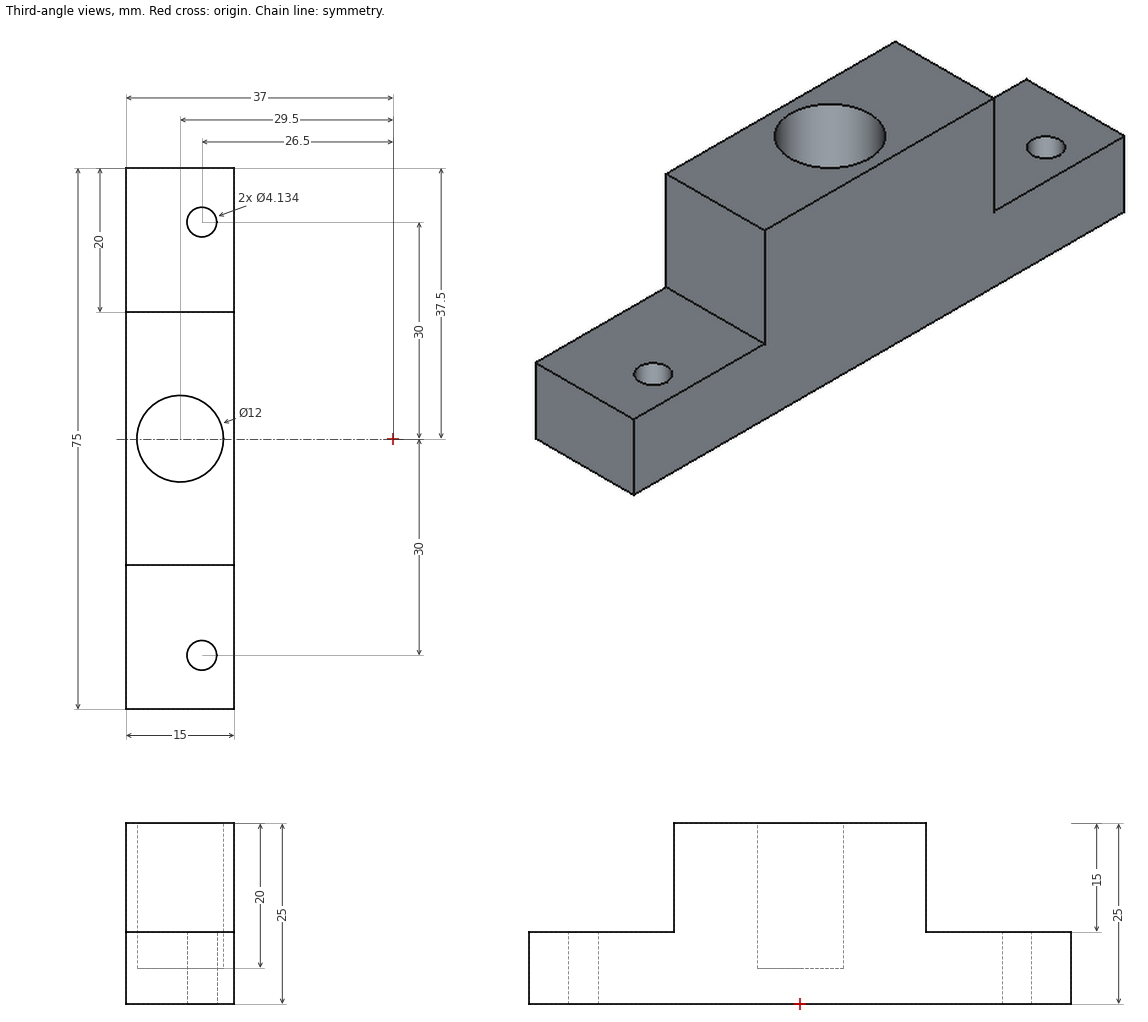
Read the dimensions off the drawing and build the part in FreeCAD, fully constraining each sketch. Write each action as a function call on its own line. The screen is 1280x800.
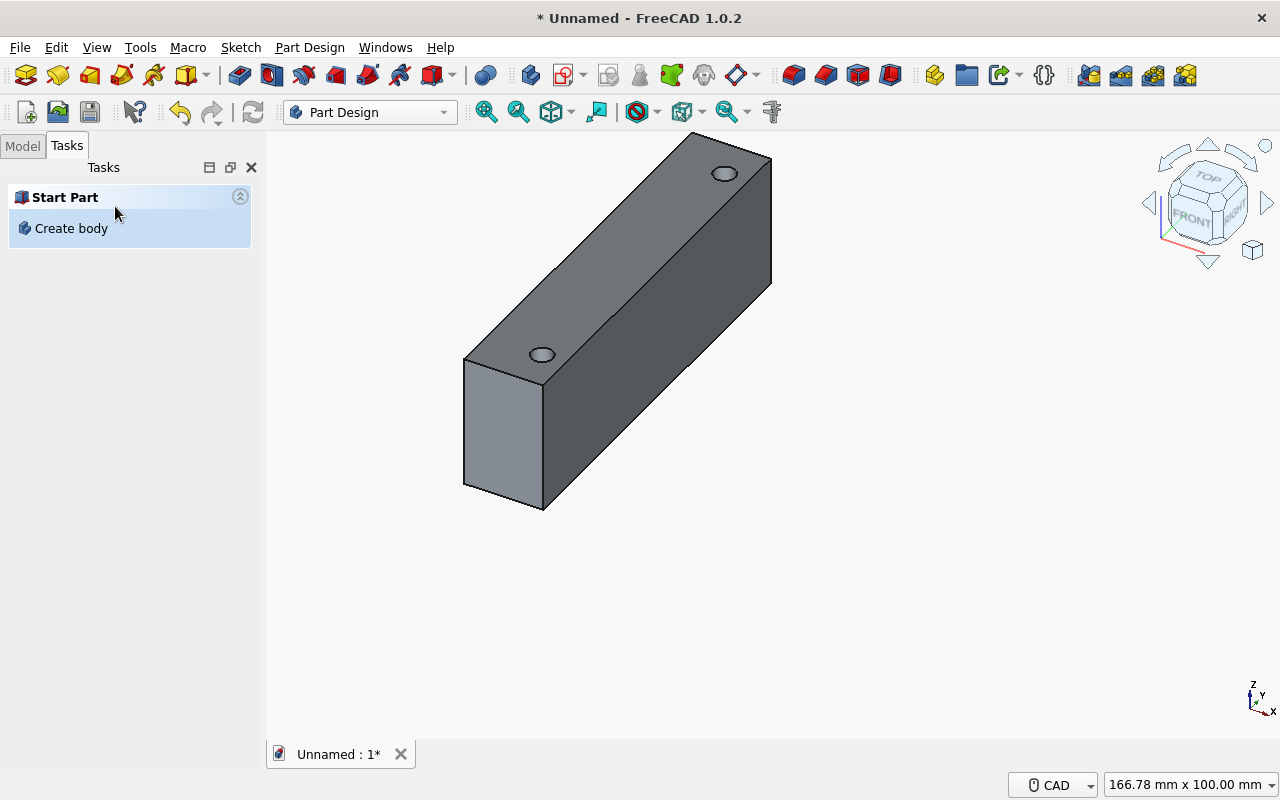
click(650, 226)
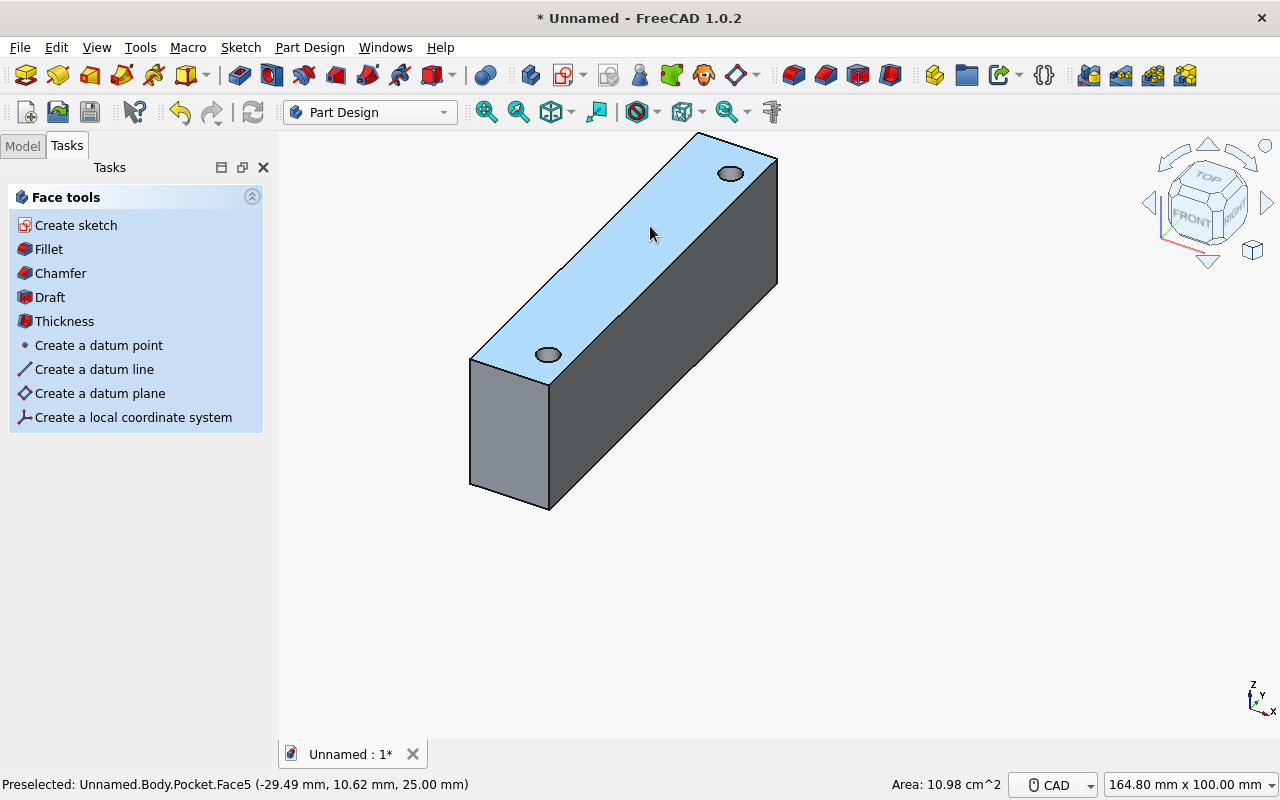
click(564, 76)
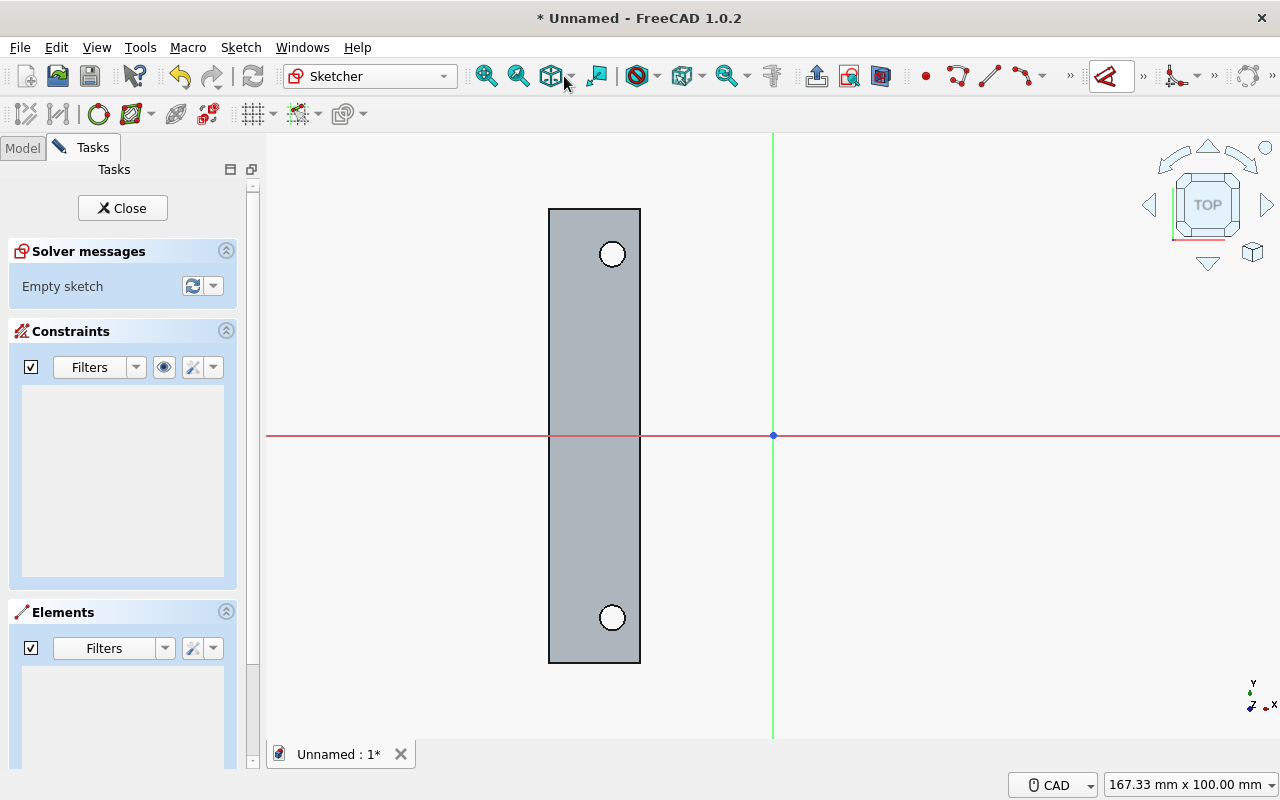
key(g)
key(r)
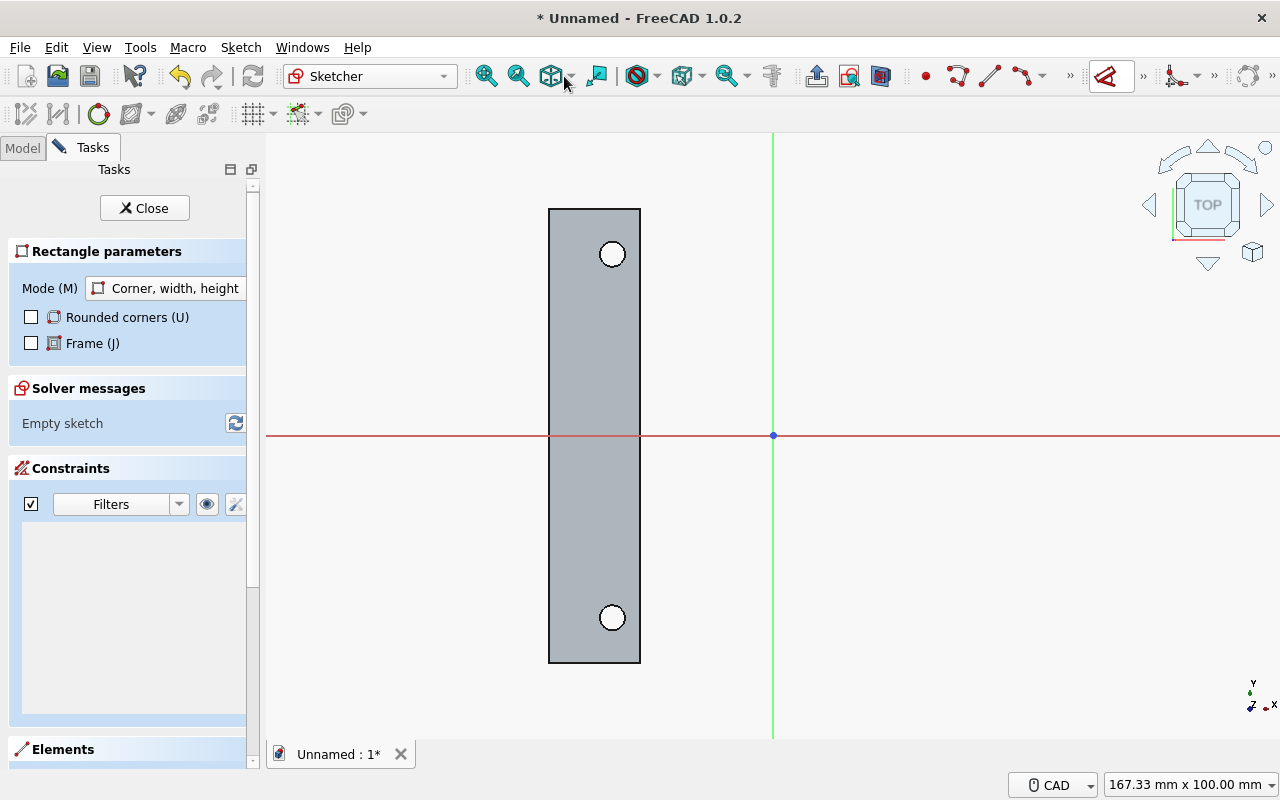
click(549, 209)
click(640, 330)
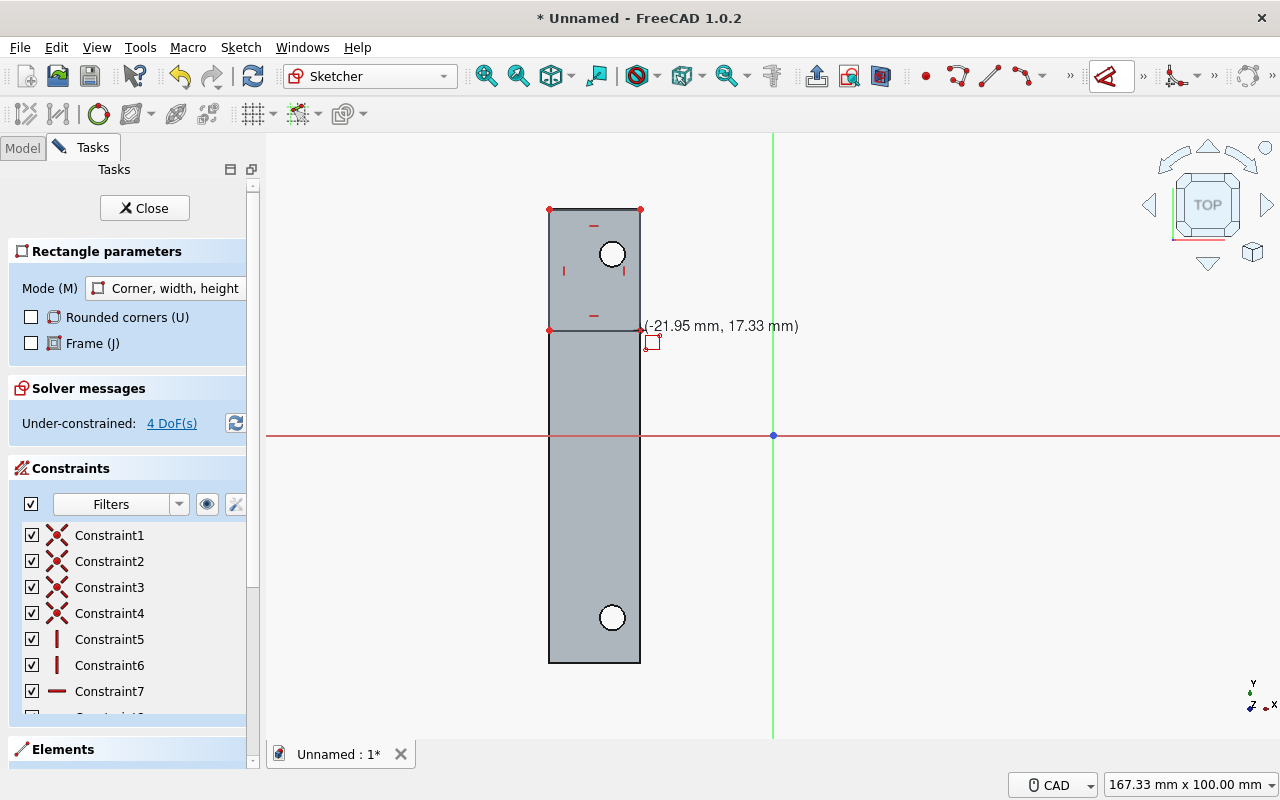
click(549, 542)
click(640, 663)
key(Escape)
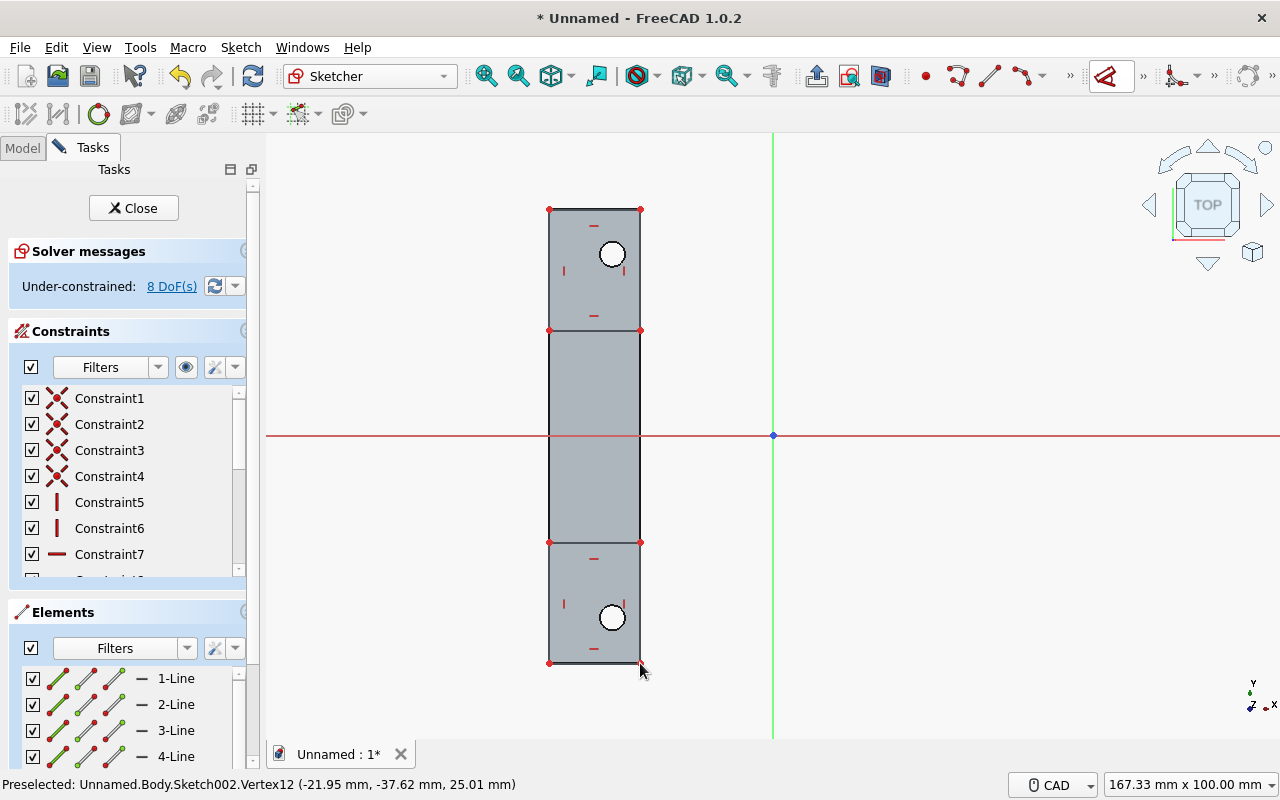
click(549, 331)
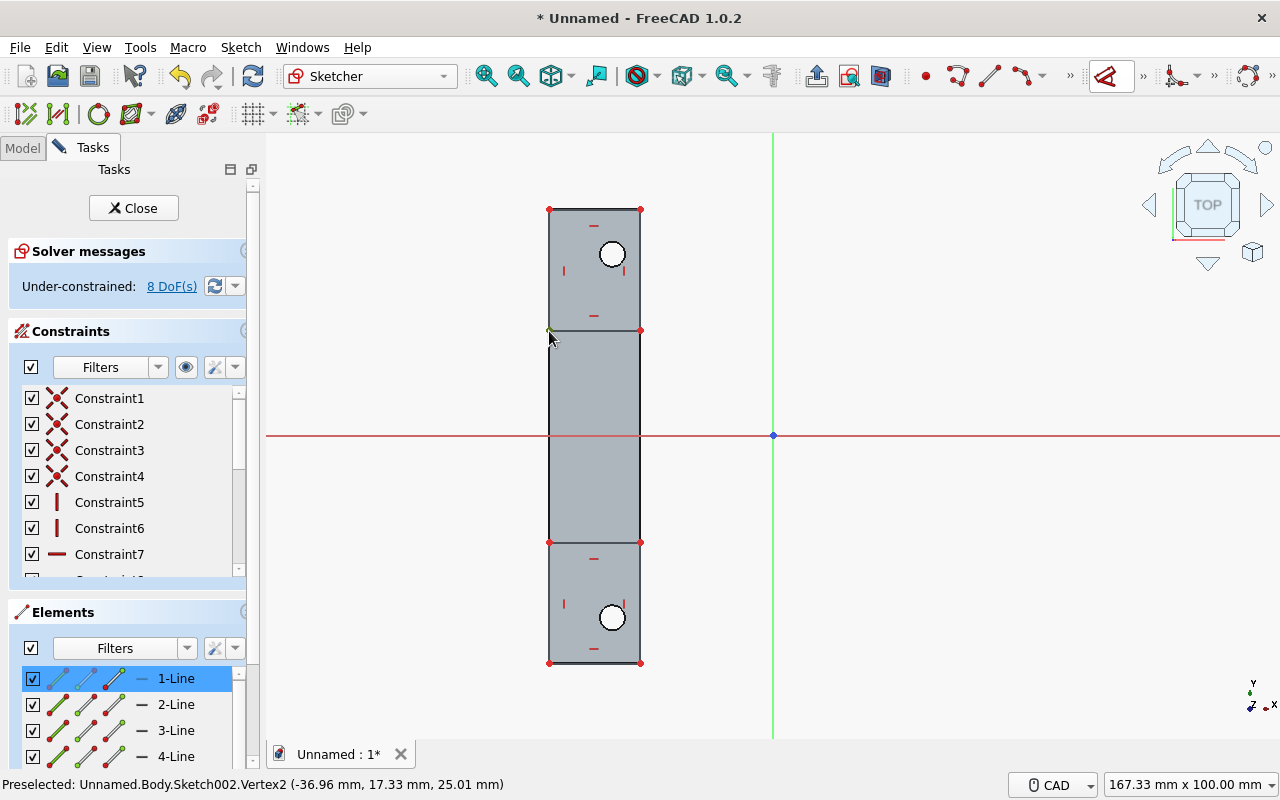
click(549, 543)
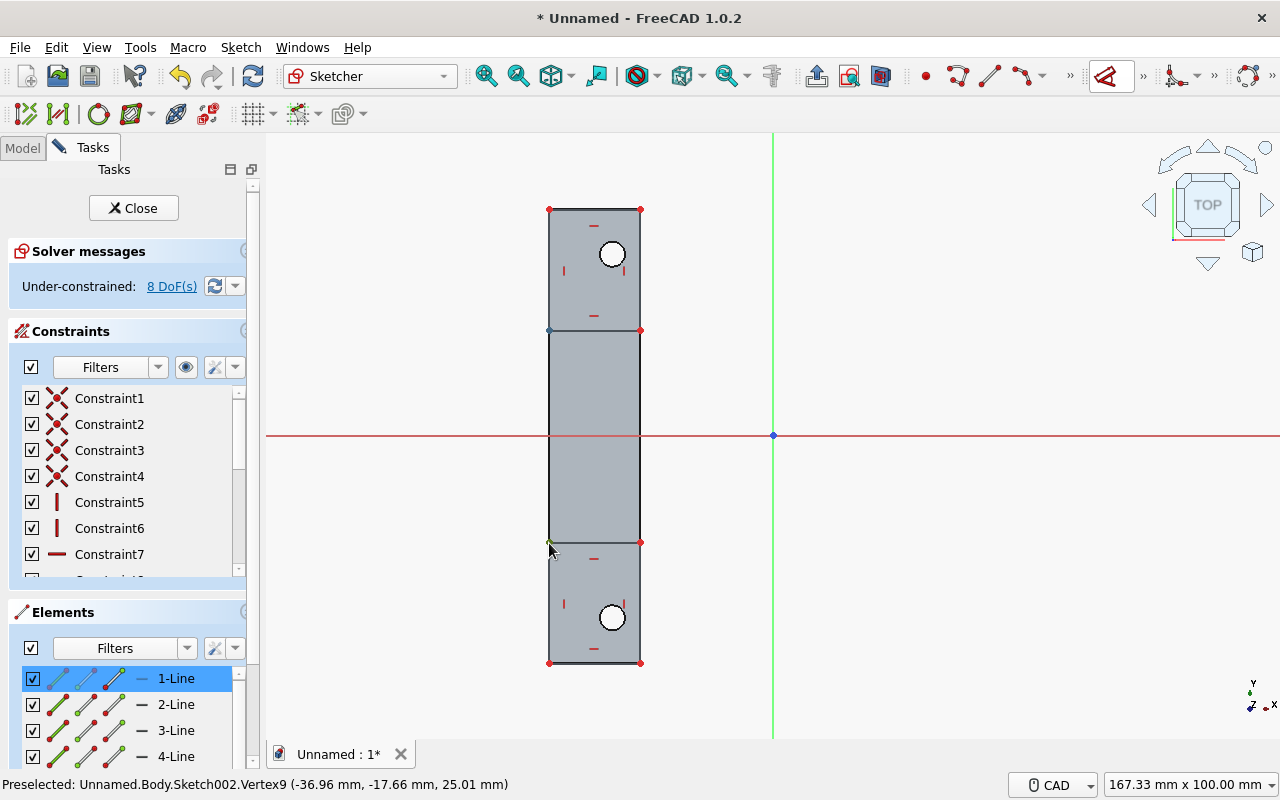
click(353, 436)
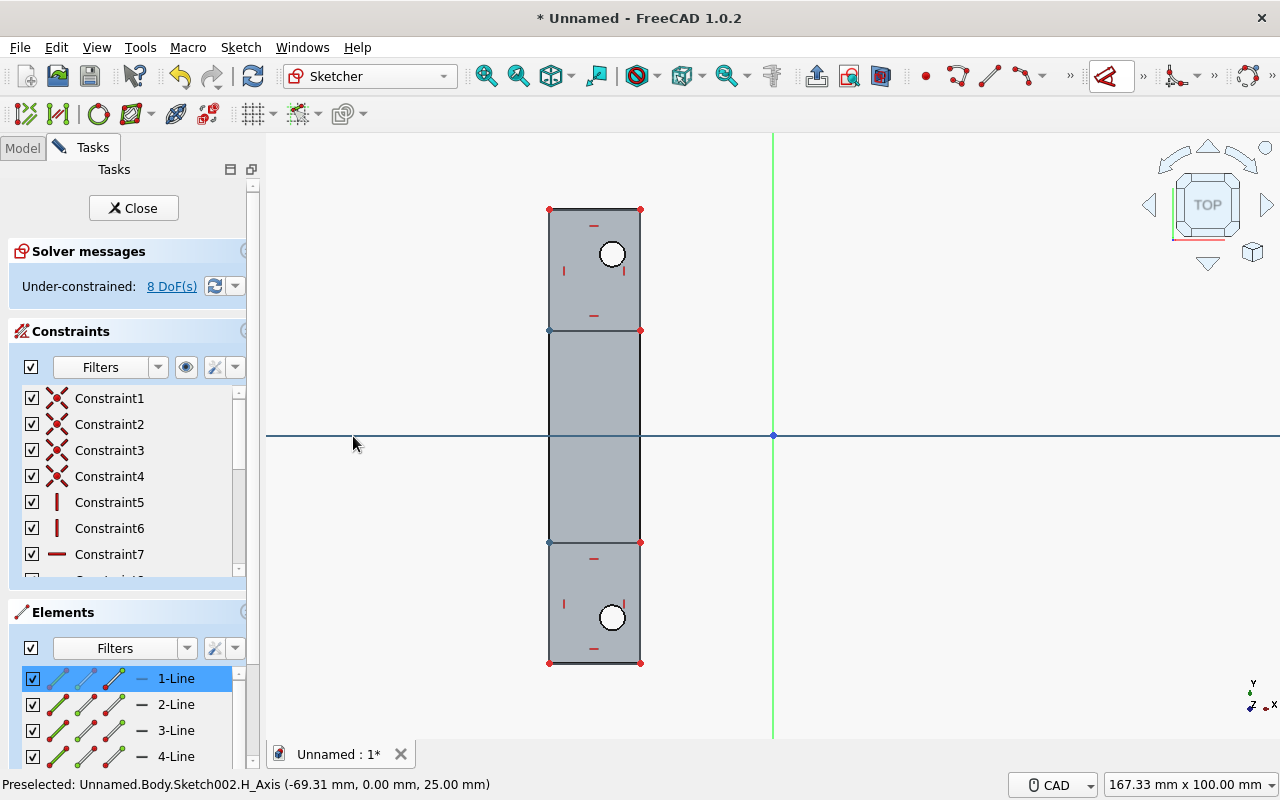
key(s)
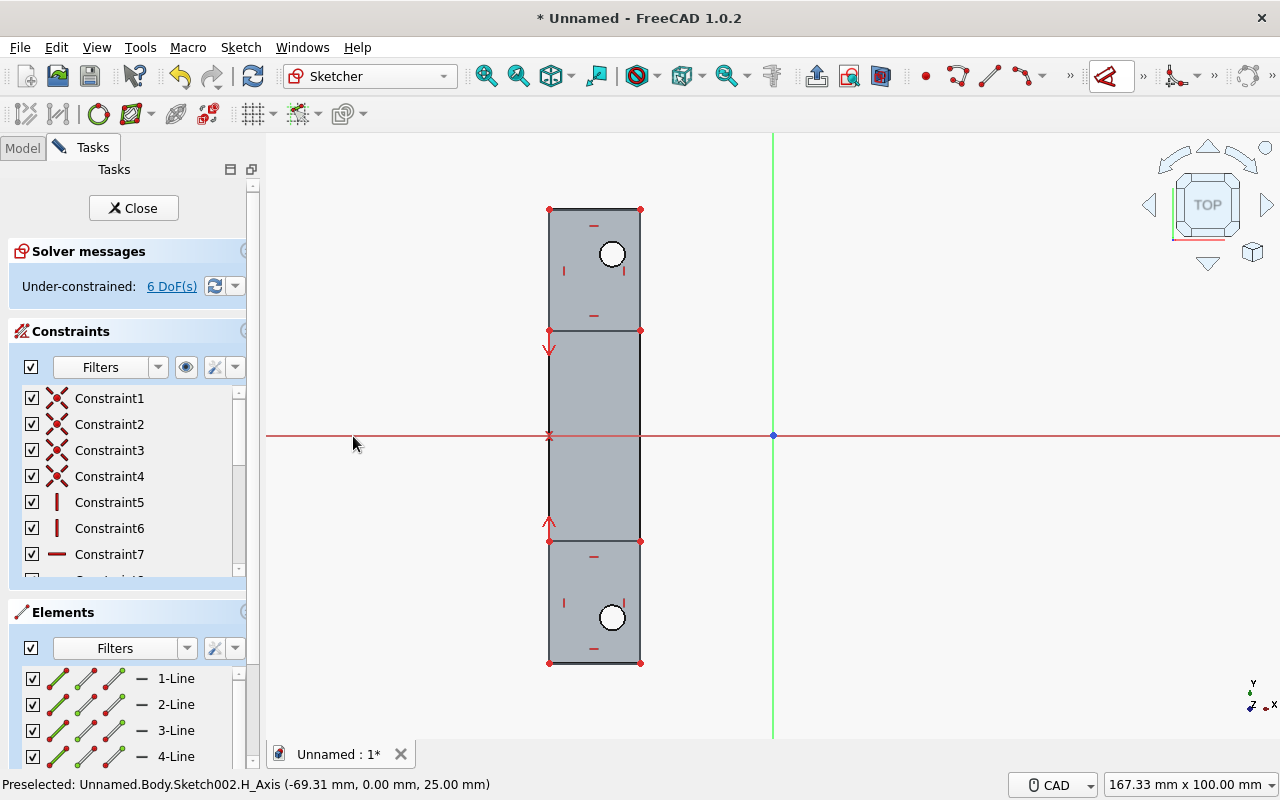
click(640, 210)